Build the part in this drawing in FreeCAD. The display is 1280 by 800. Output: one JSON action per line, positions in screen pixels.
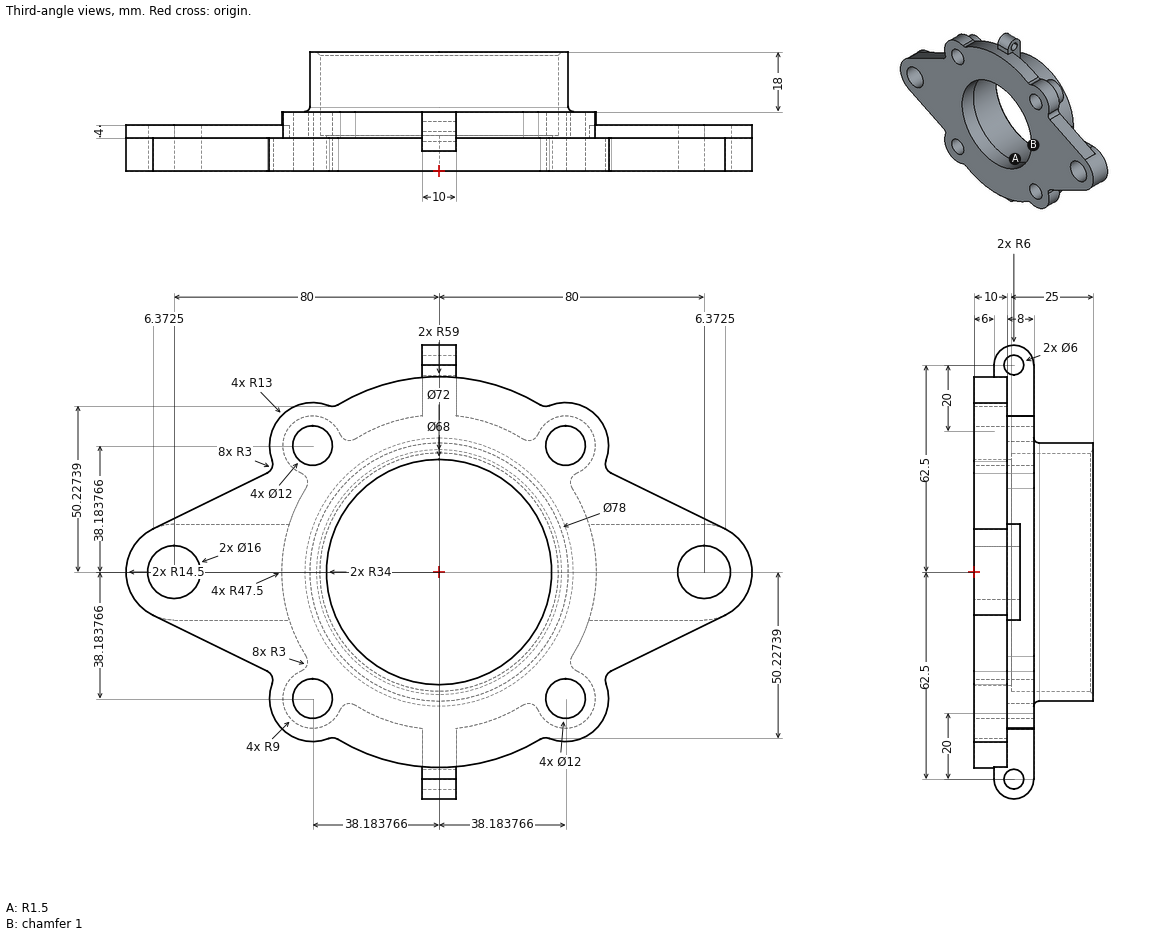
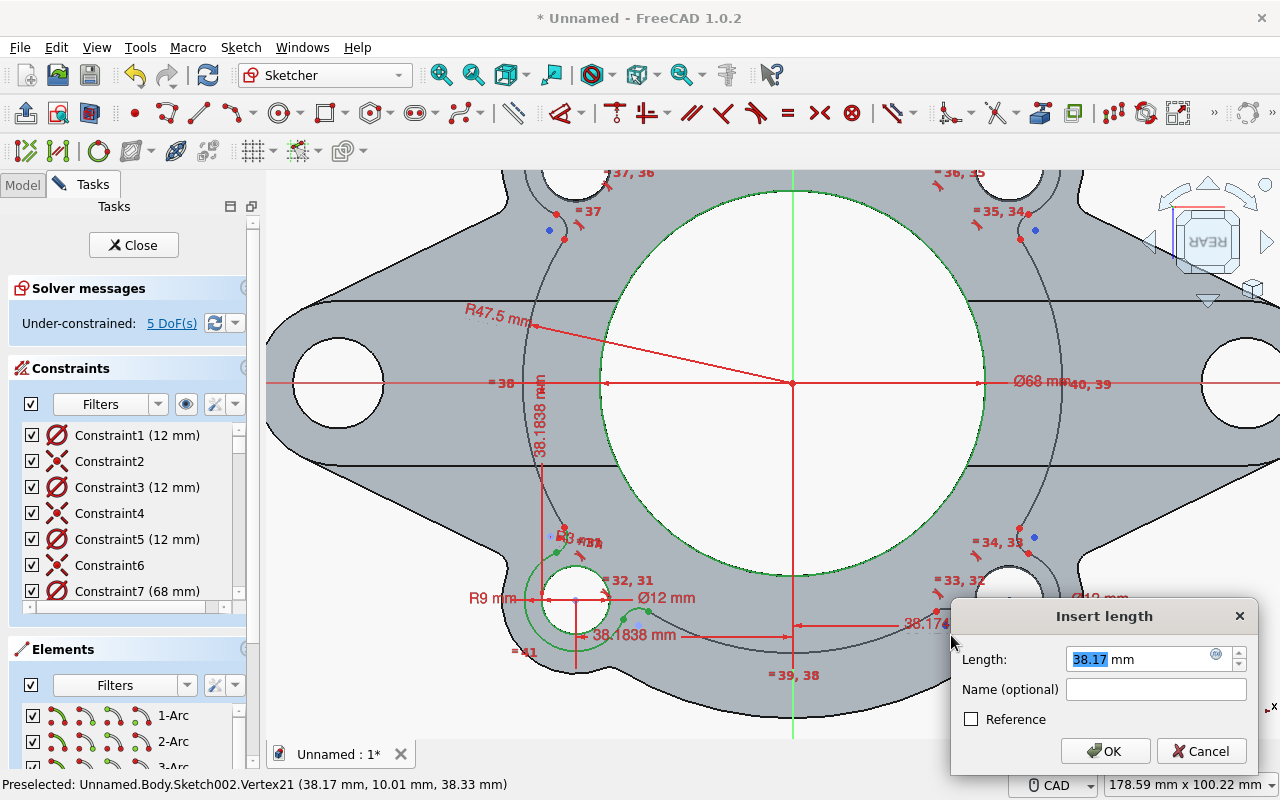
{"action": "type", "text": "38.183766"}
{"action": "key", "text": "Return"}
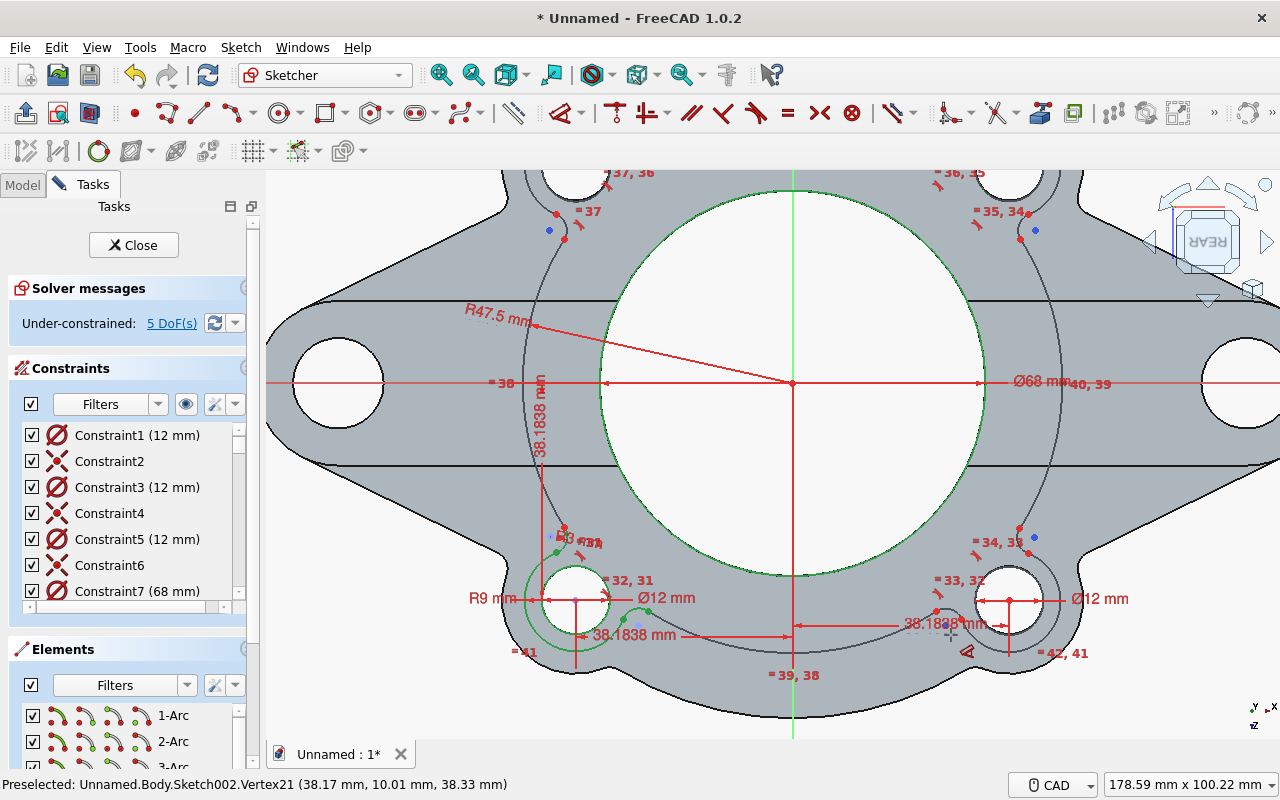
{"action": "left_click", "coordinate": [1009, 601]}
{"action": "left_click", "coordinate": [1043, 542]}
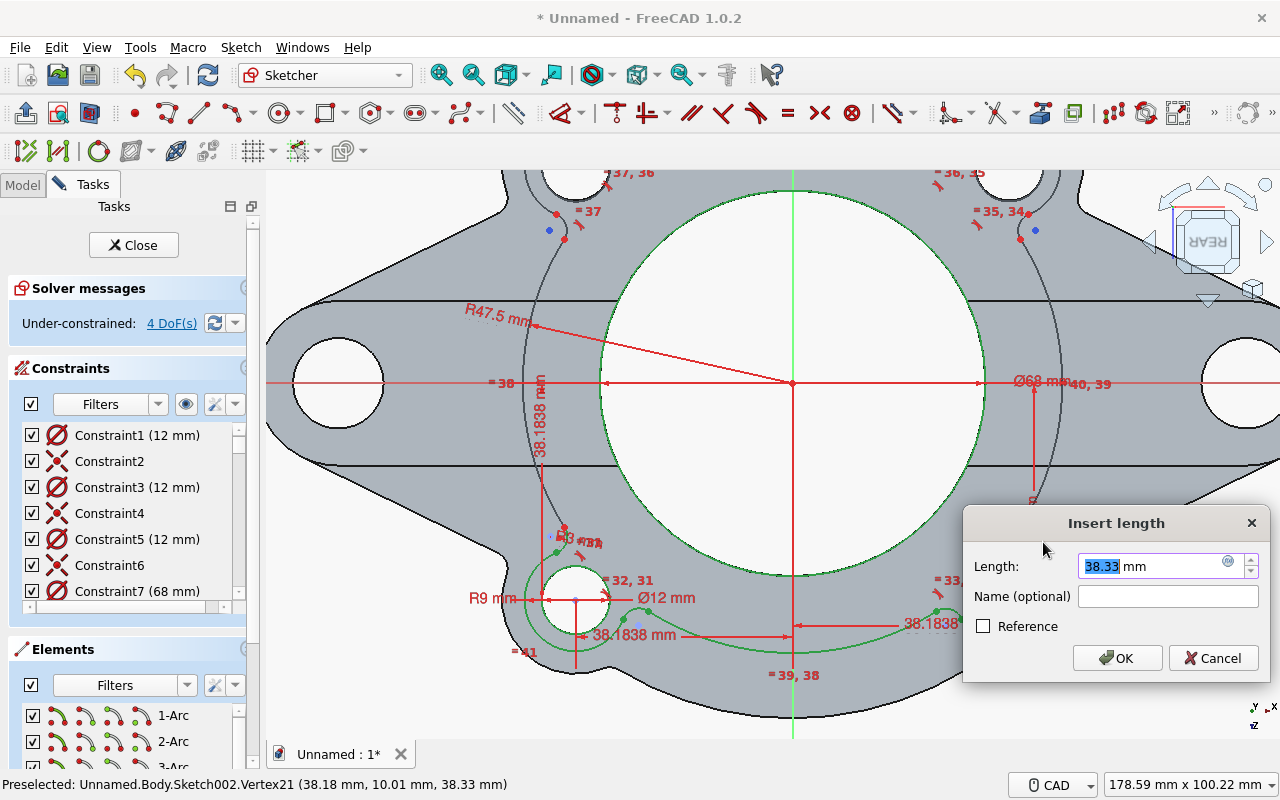
{"action": "type", "text": "38.183766"}
{"action": "key", "text": "Return"}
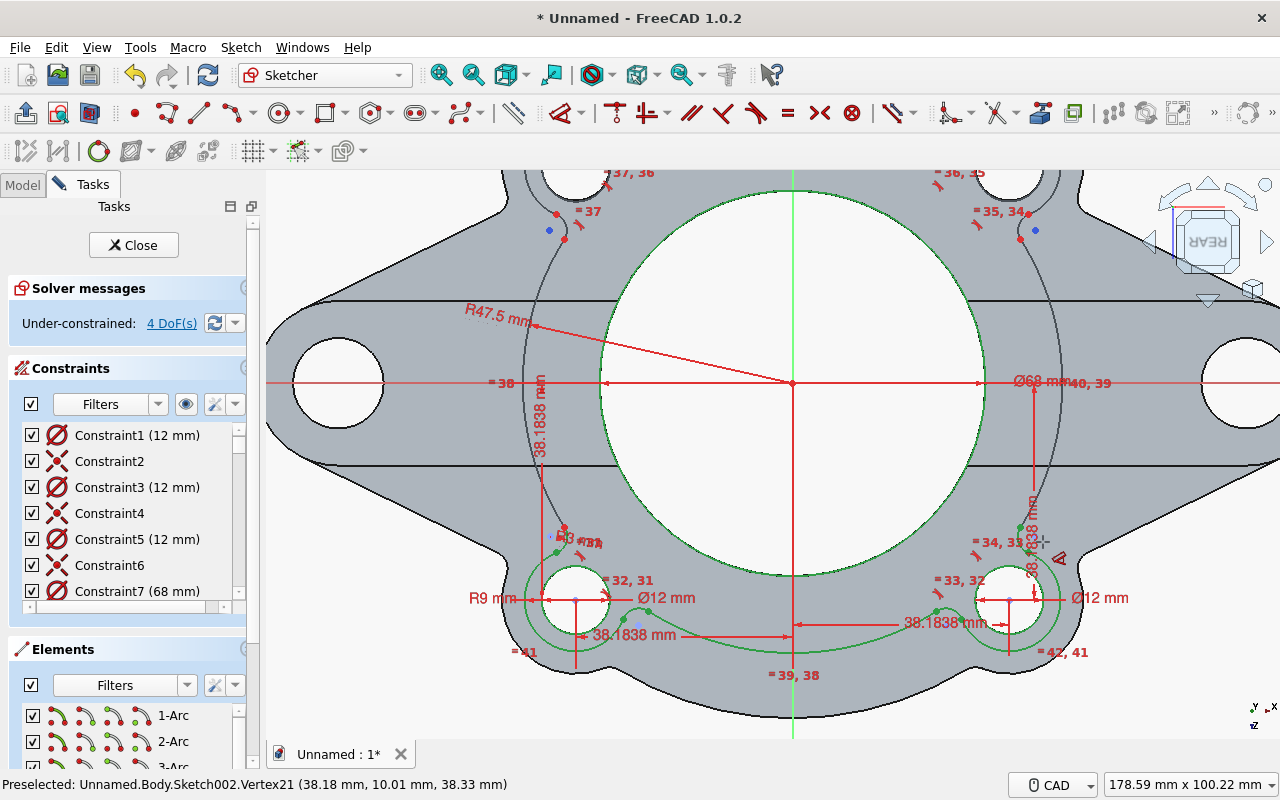
{"action": "scroll", "coordinate": [525, 599], "scroll_direction": "down", "scroll_amount": 2}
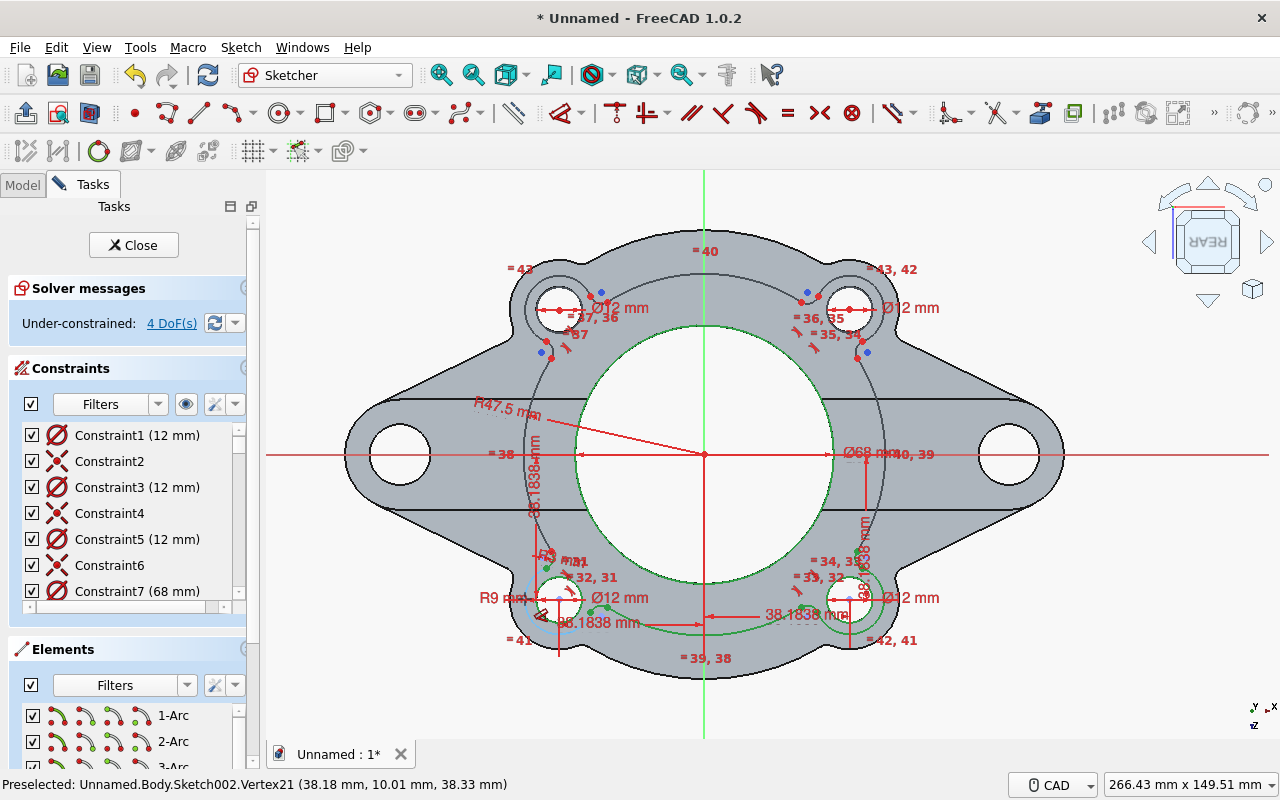
{"action": "left_click", "coordinate": [559, 310]}
{"action": "left_click", "coordinate": [599, 276]}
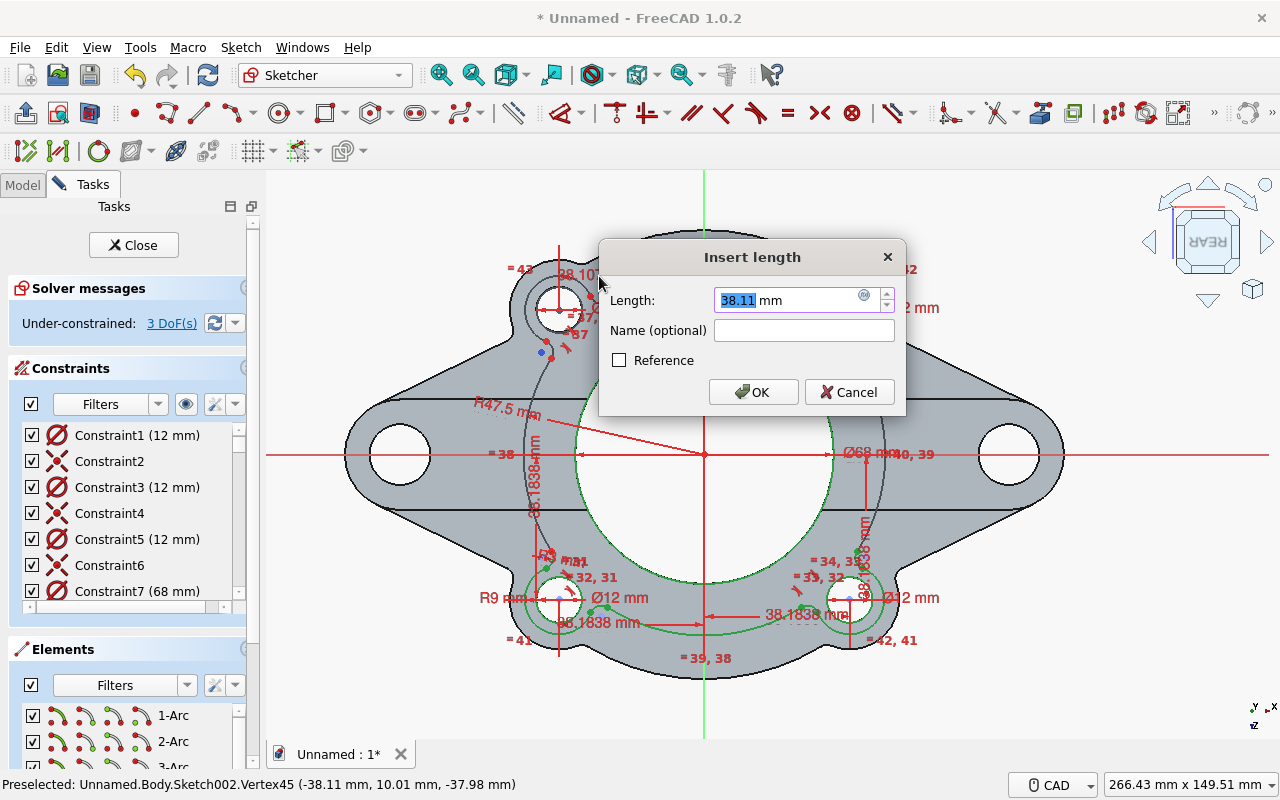
{"action": "type", "text": "38.183766"}
{"action": "key", "text": "Return"}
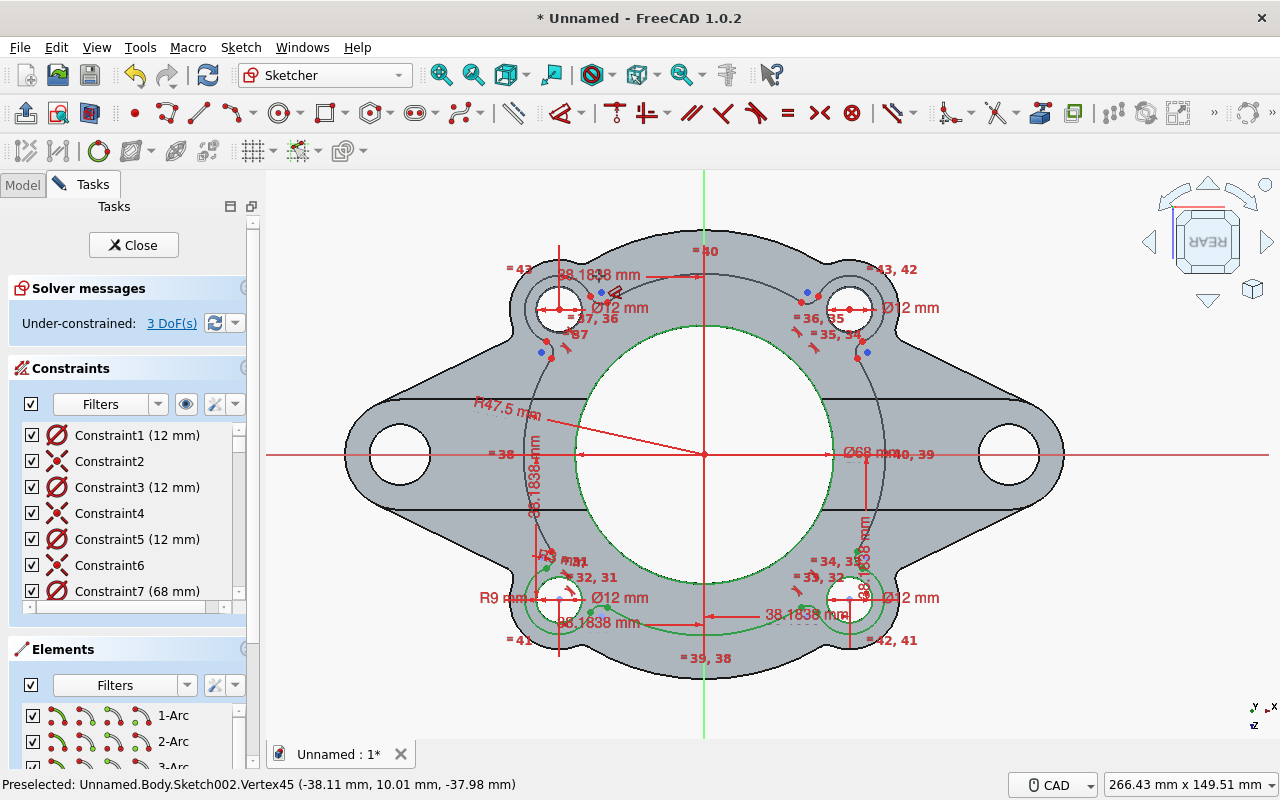
{"action": "left_click", "coordinate": [559, 310]}
{"action": "left_click", "coordinate": [525, 349]}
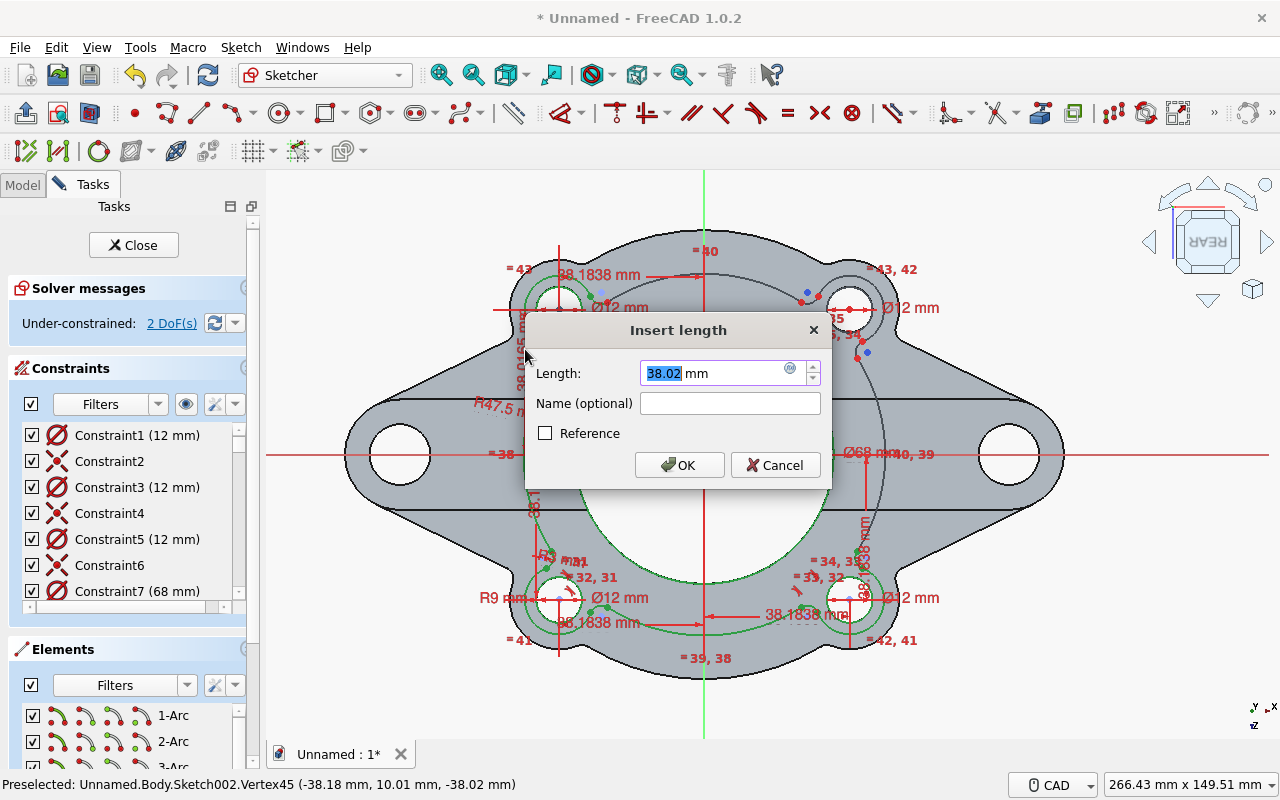
{"action": "type", "text": "38.183766"}
{"action": "key", "text": "Return"}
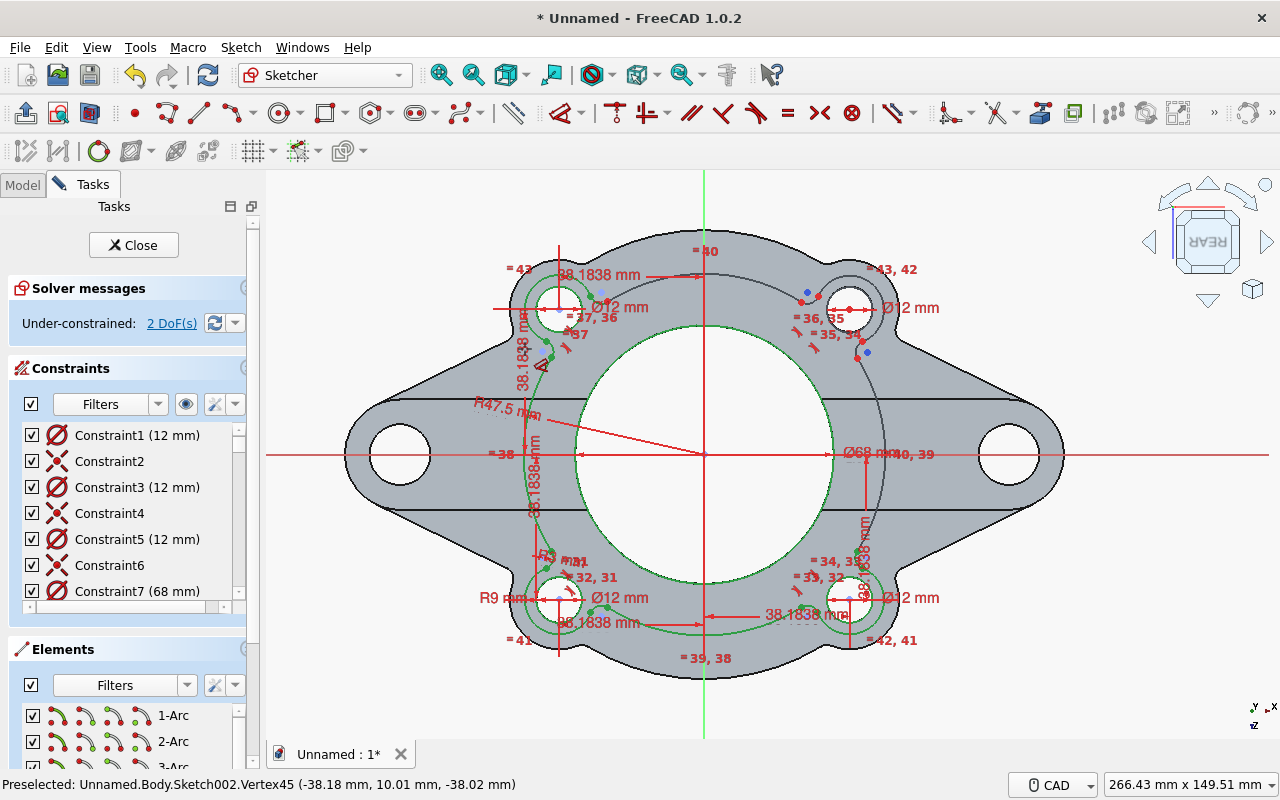
{"action": "left_click", "coordinate": [850, 310]}
{"action": "left_click", "coordinate": [810, 276]}